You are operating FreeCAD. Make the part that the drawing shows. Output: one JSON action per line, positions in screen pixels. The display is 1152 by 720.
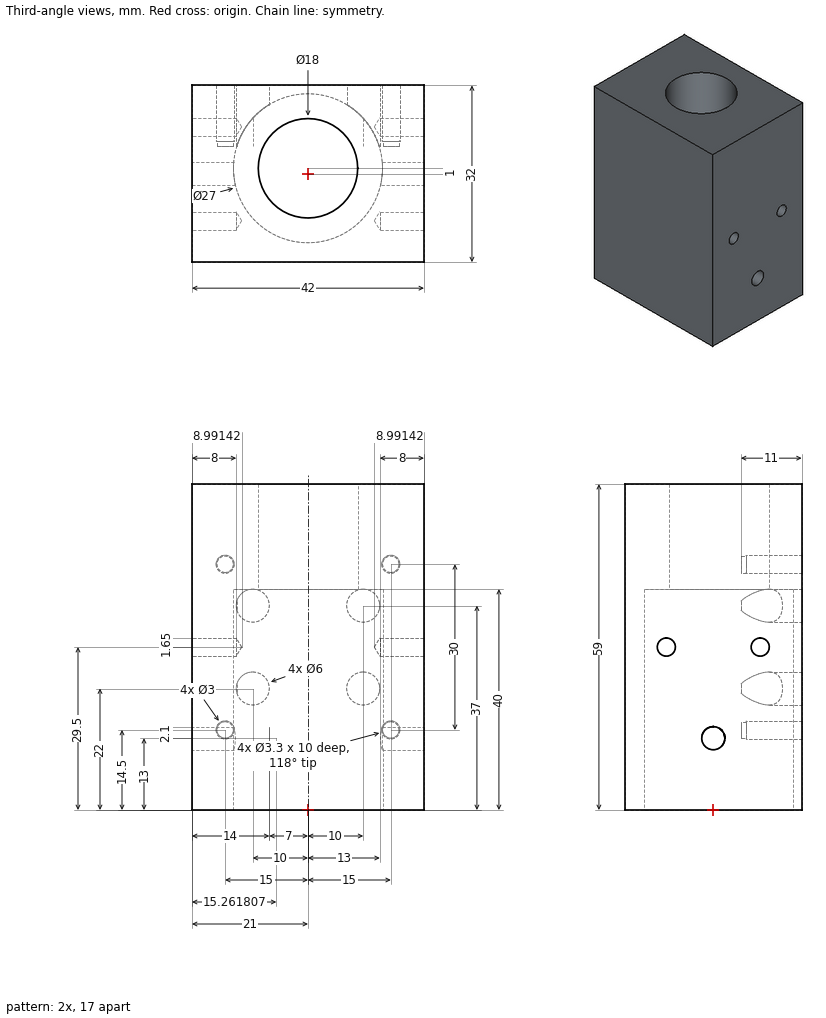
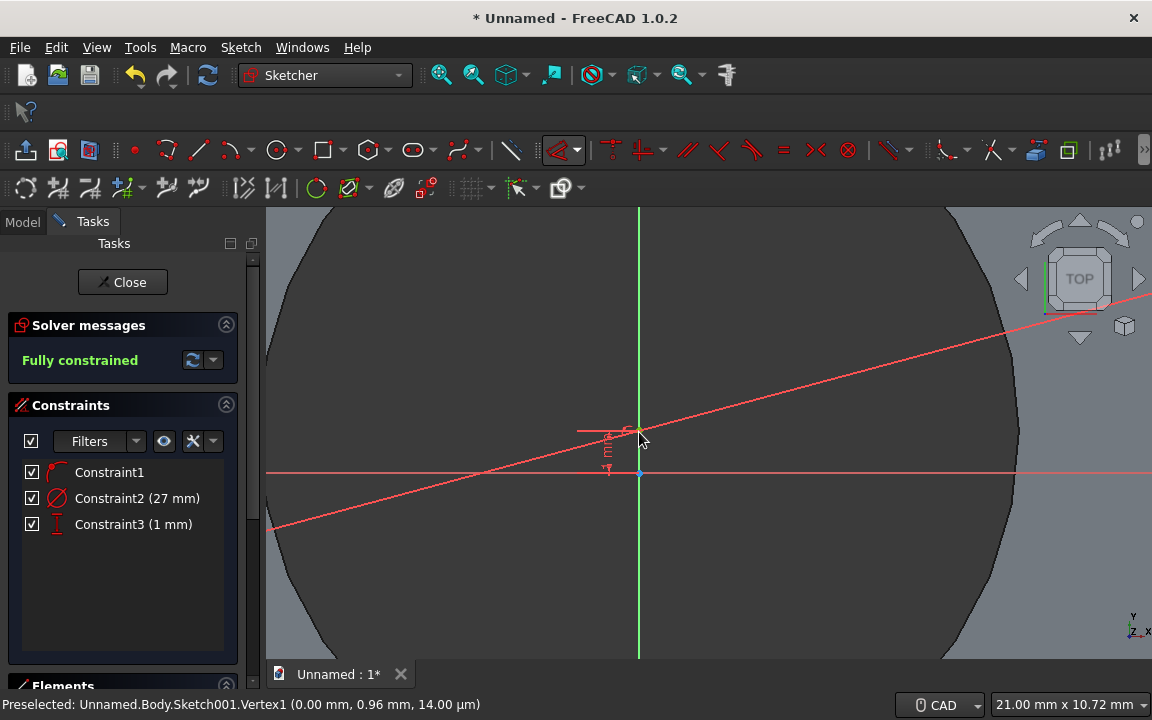
{"action": "left_click", "coordinate": [123, 282]}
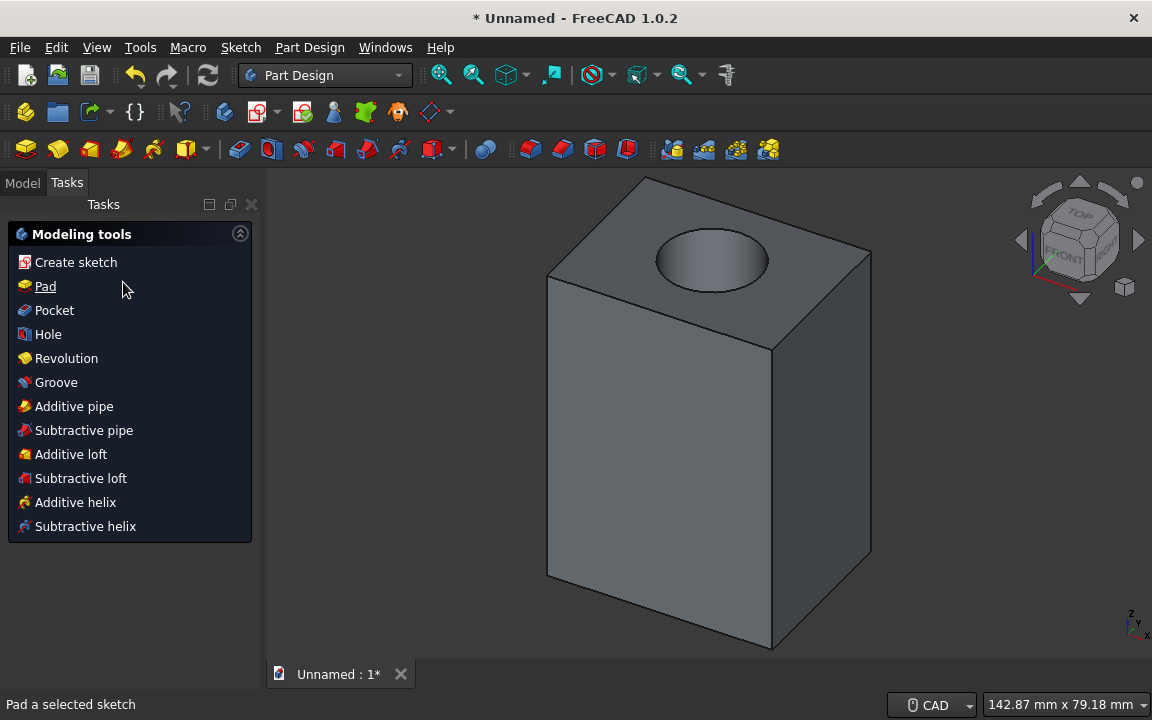
{"action": "left_click", "coordinate": [240, 150]}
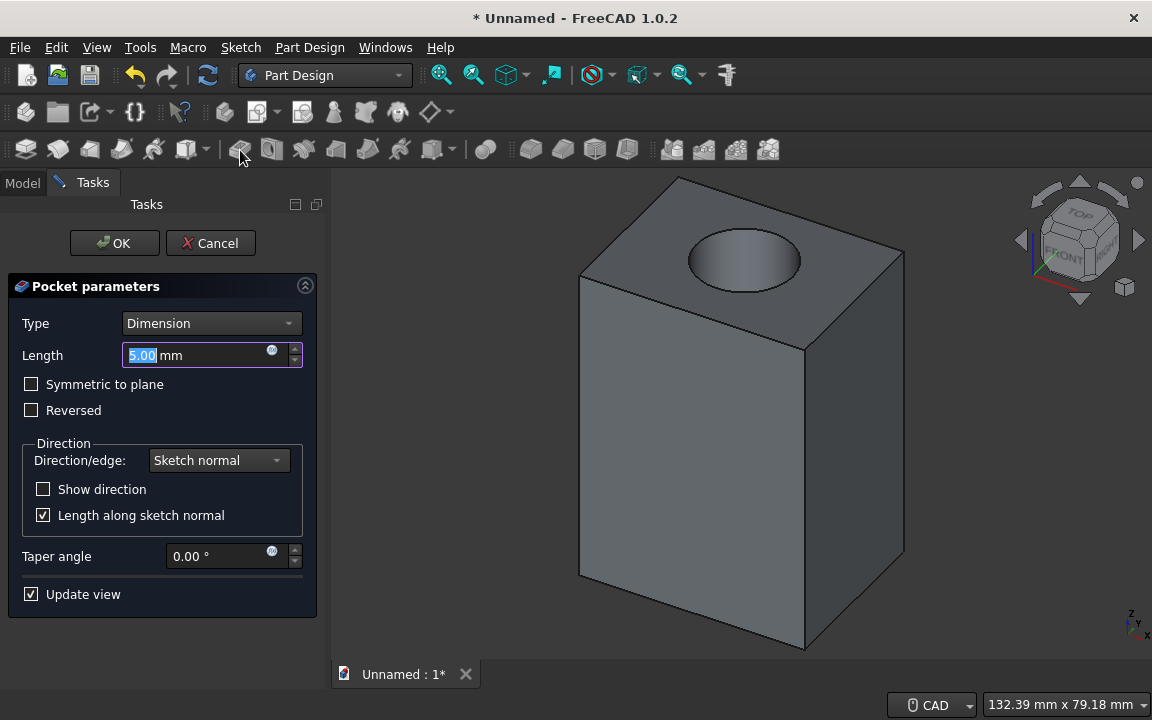
{"action": "type", "text": "40"}
{"action": "key", "text": "Tab"}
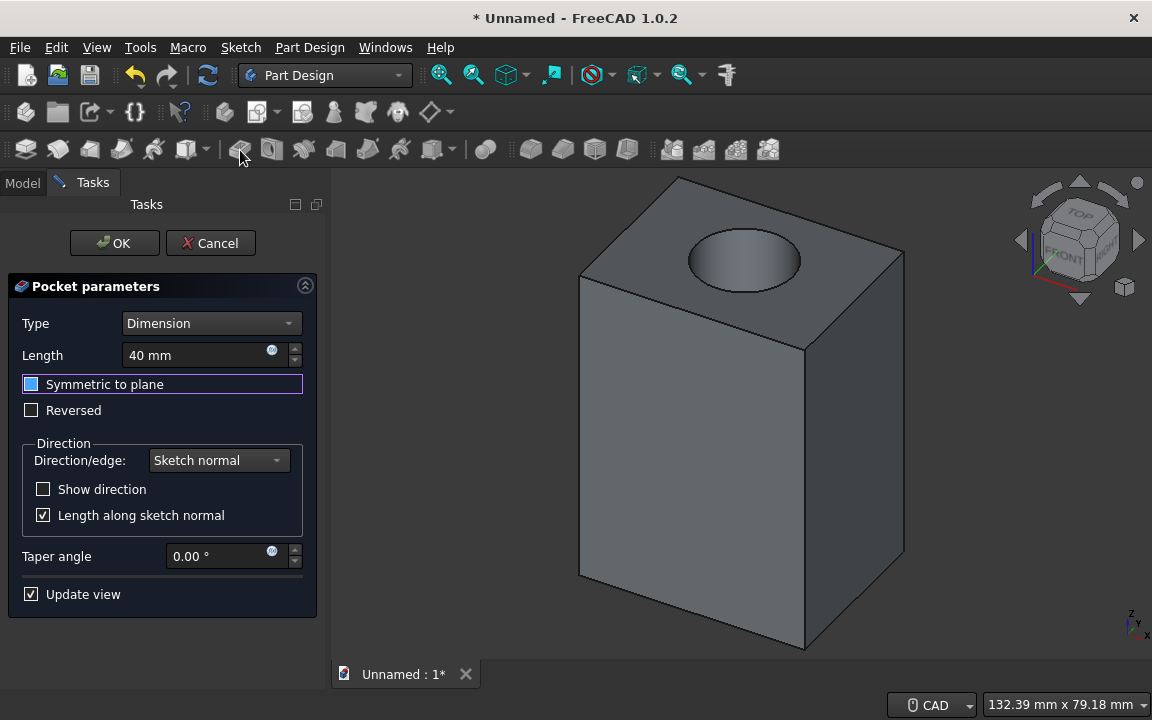
{"action": "left_click", "coordinate": [30, 410]}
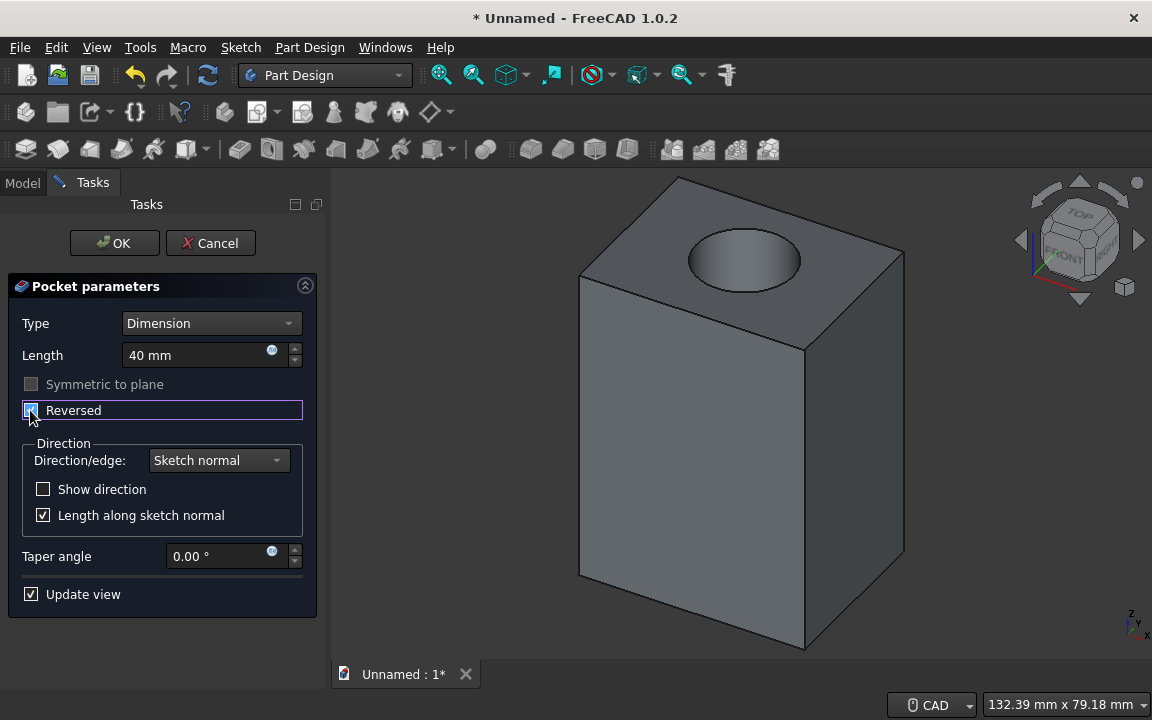
{"action": "left_click", "coordinate": [115, 243]}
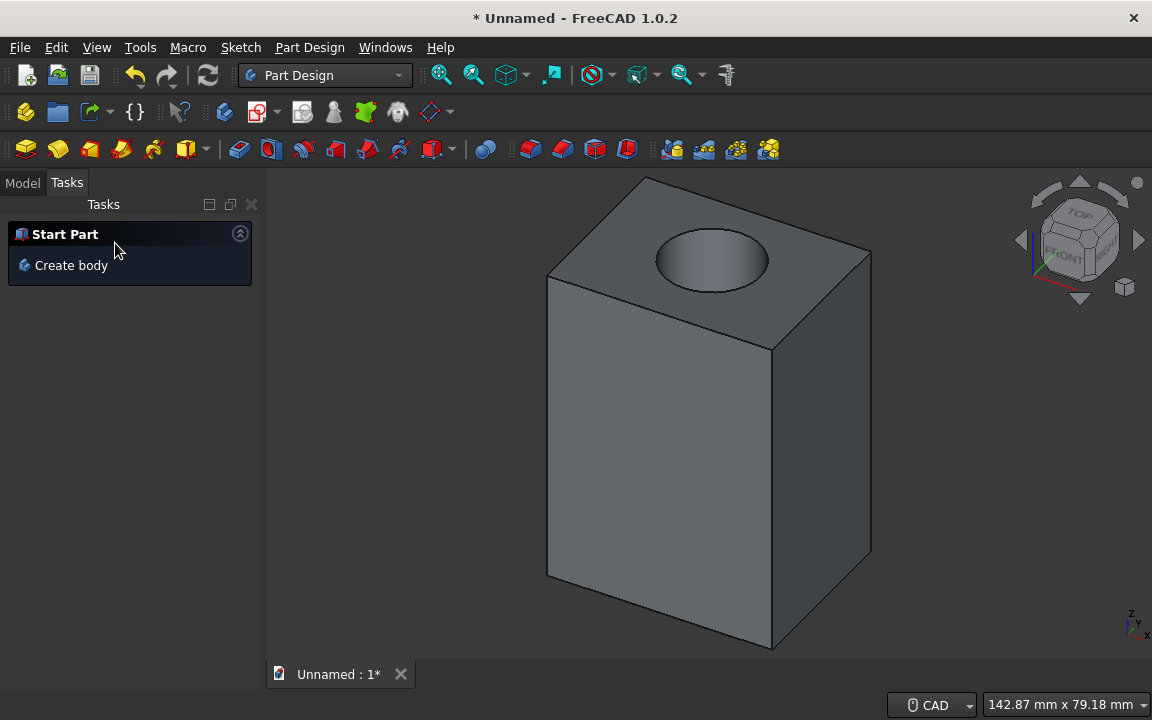
{"action": "left_click", "coordinate": [23, 182]}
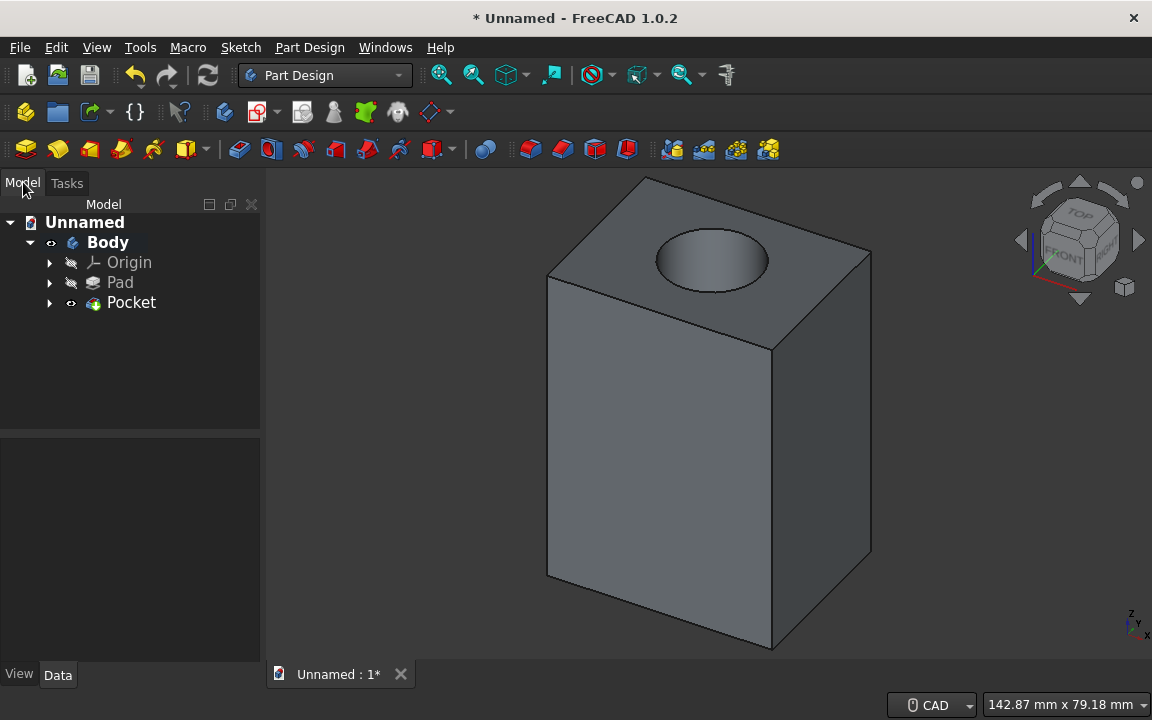
{"action": "left_click", "coordinate": [50, 263]}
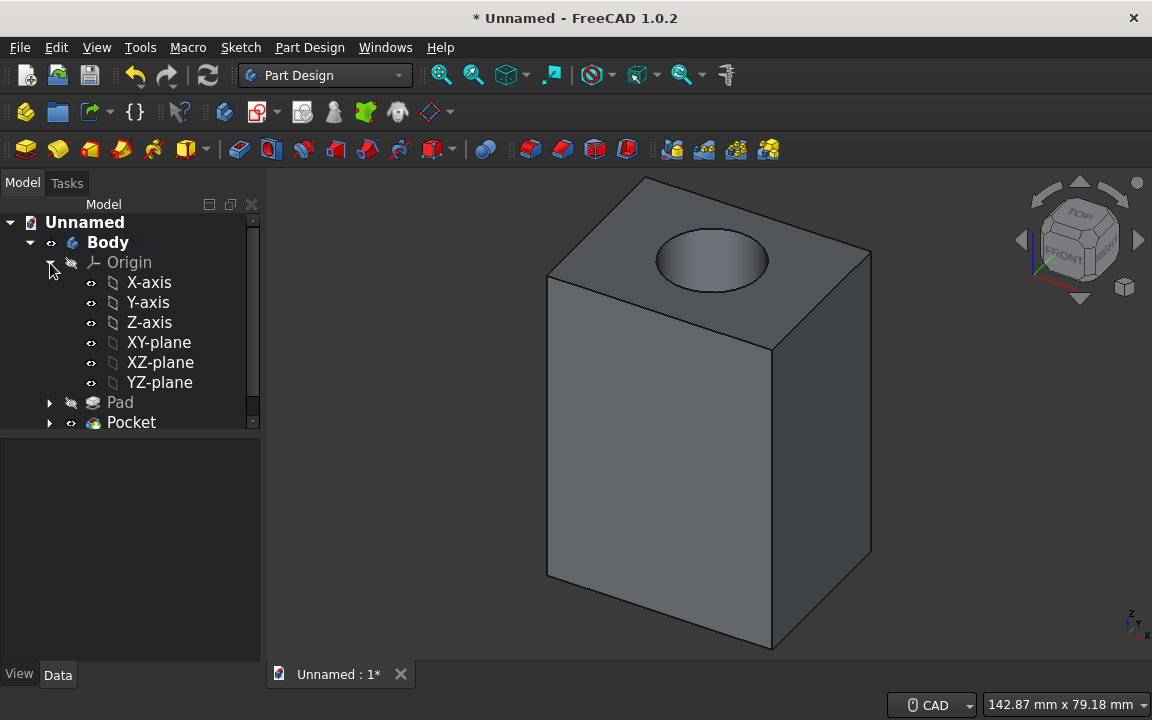
{"action": "left_click", "coordinate": [136, 363]}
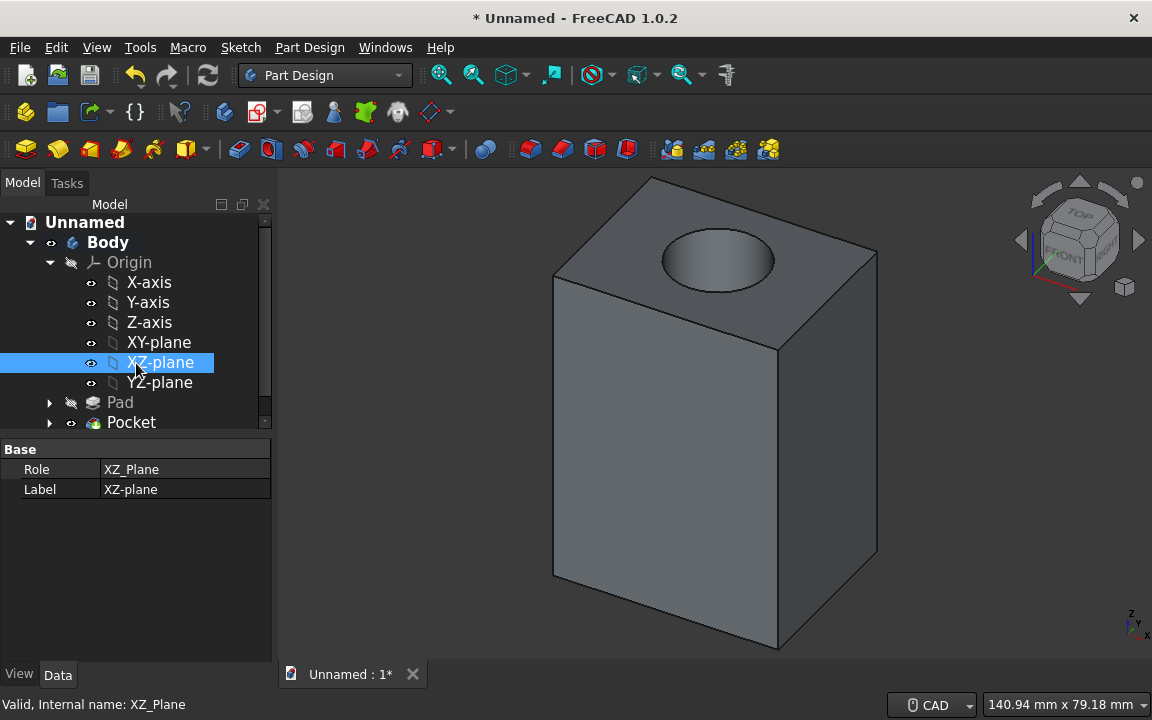
{"action": "left_click", "coordinate": [430, 112]}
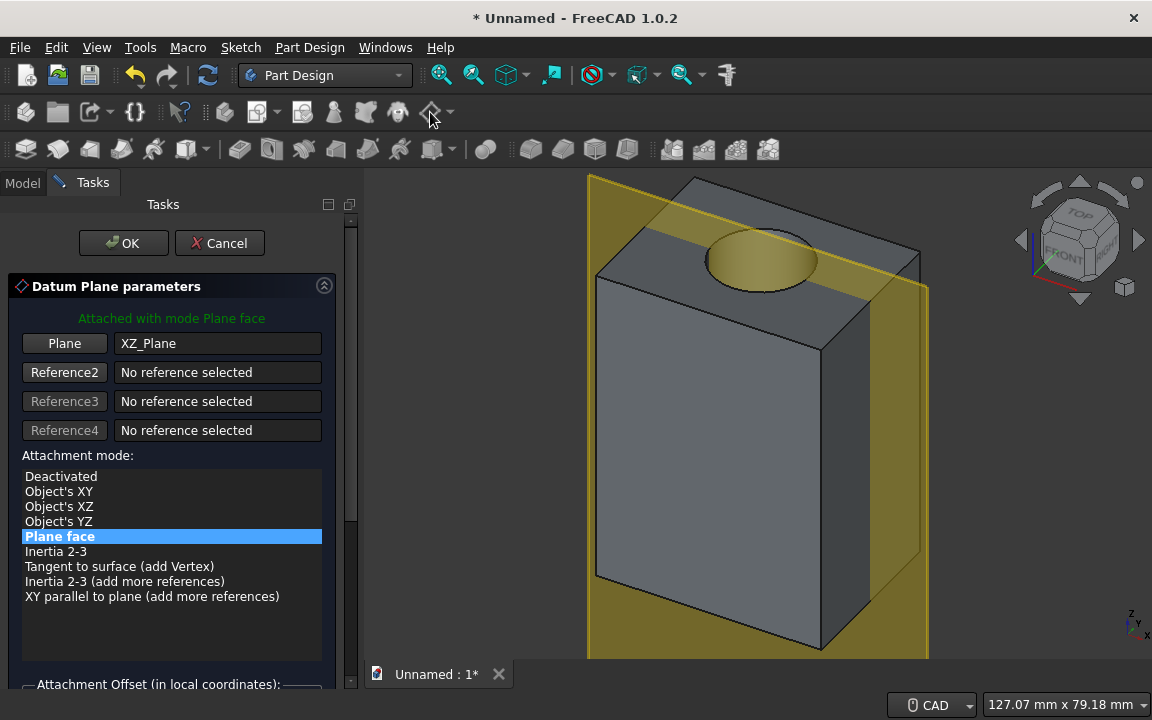
{"action": "scroll", "coordinate": [351, 451], "scroll_direction": "down", "scroll_amount": 3}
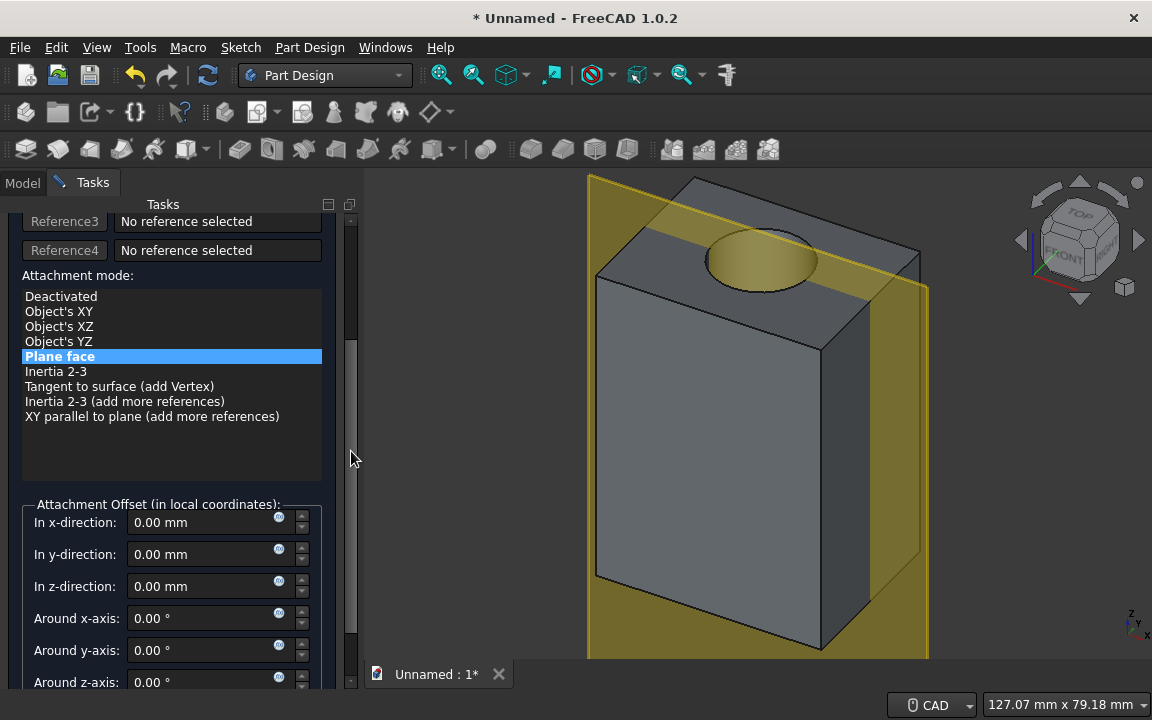
{"action": "triple_click", "coordinate": [210, 586]}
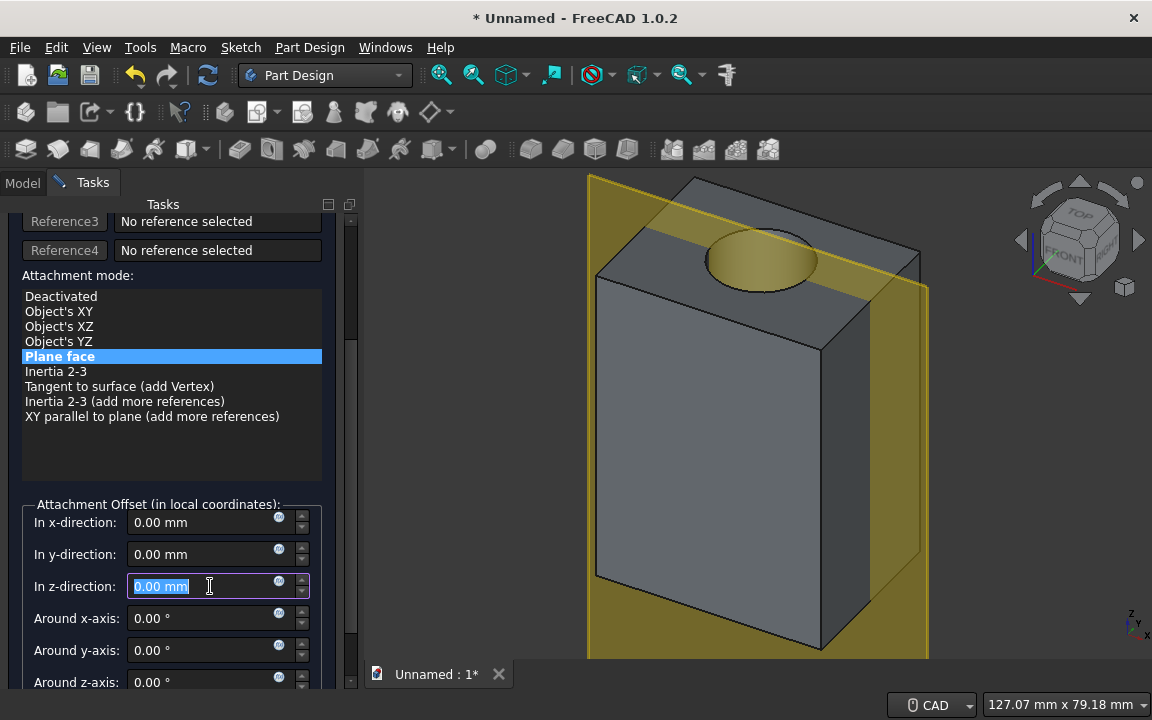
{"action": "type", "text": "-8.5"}
{"action": "key", "text": "Tab"}